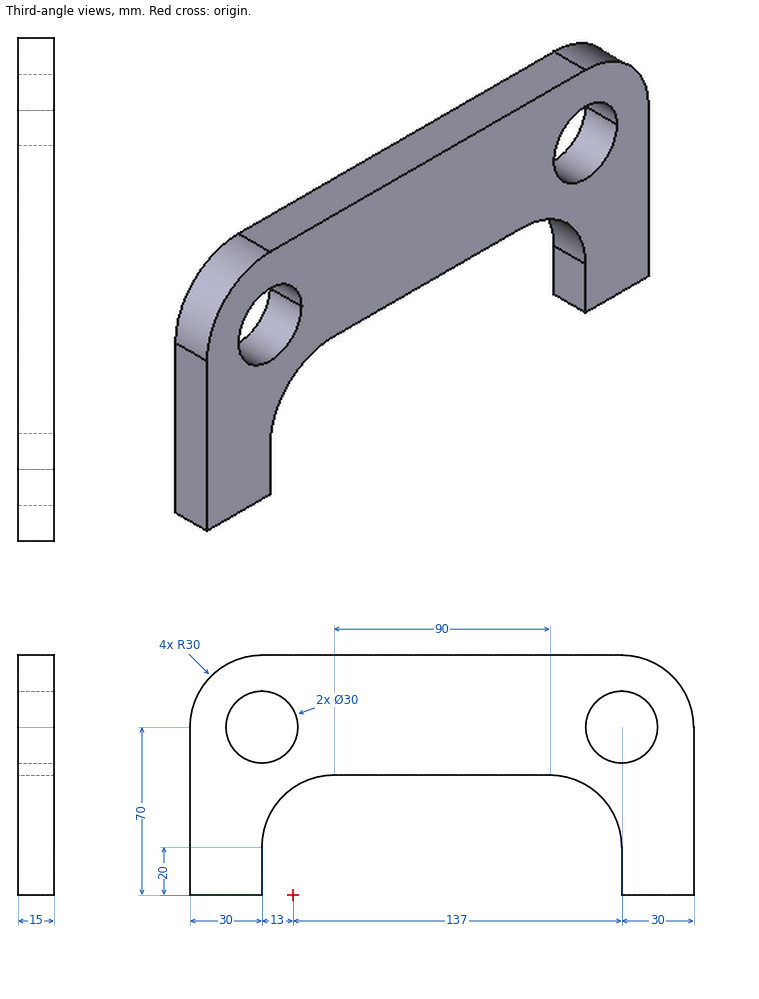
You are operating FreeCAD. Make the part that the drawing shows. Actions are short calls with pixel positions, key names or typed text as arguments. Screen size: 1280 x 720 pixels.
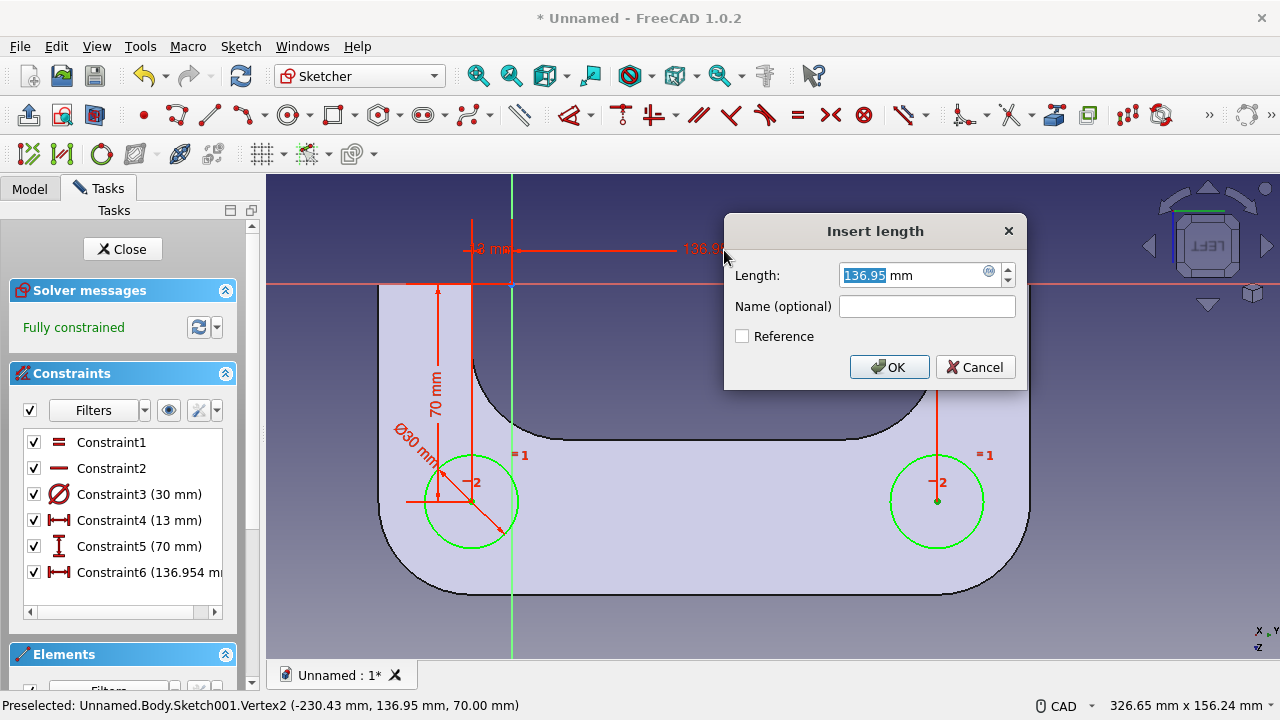
text(137)
key(Return)
key(Escape)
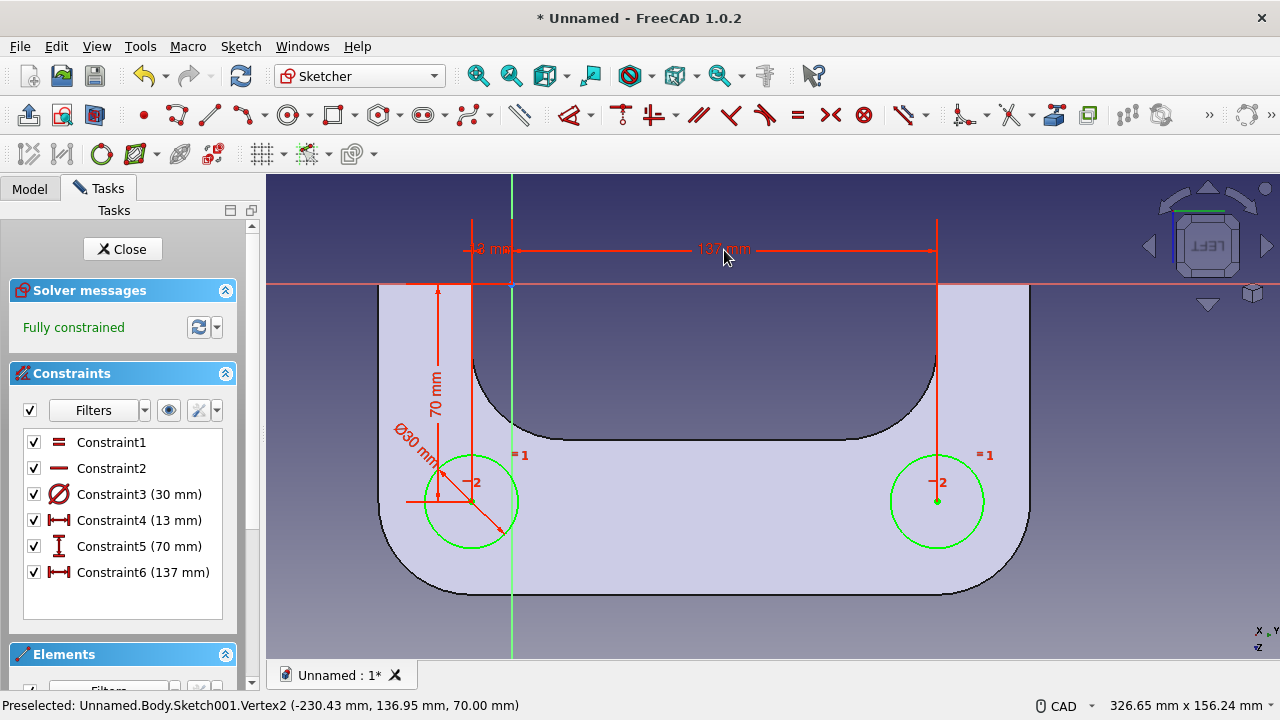
click(123, 249)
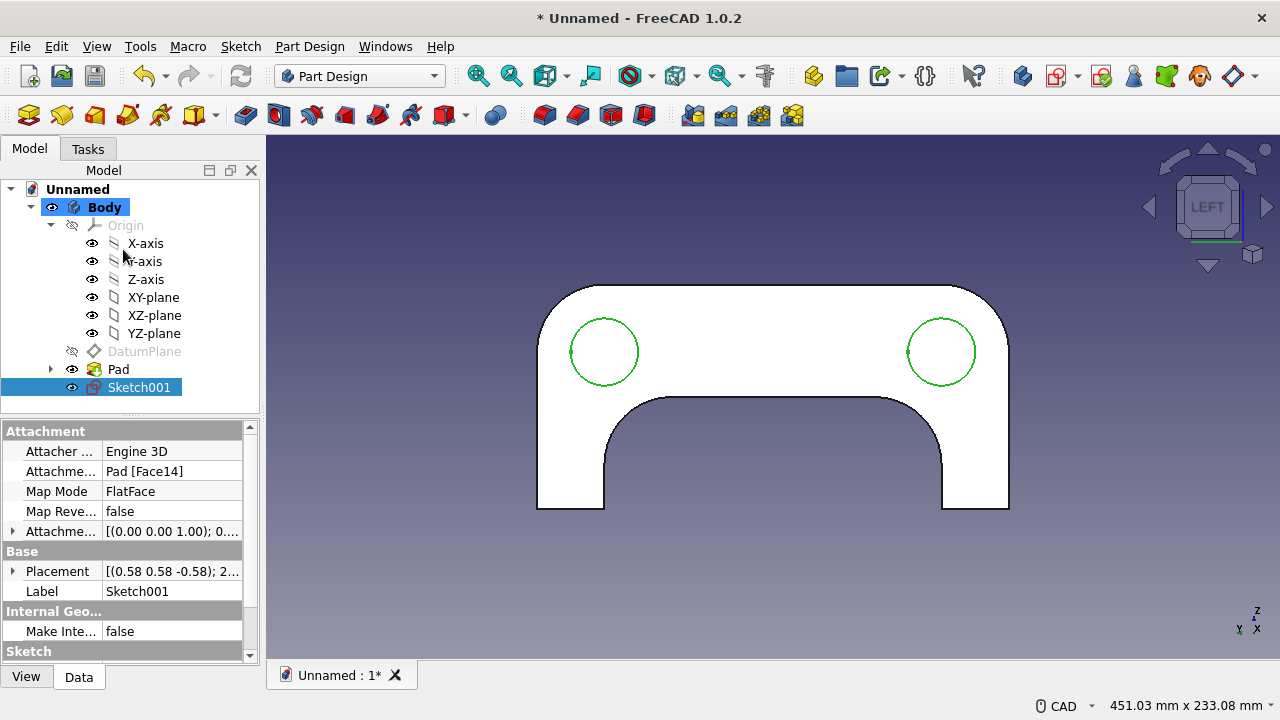
click(246, 116)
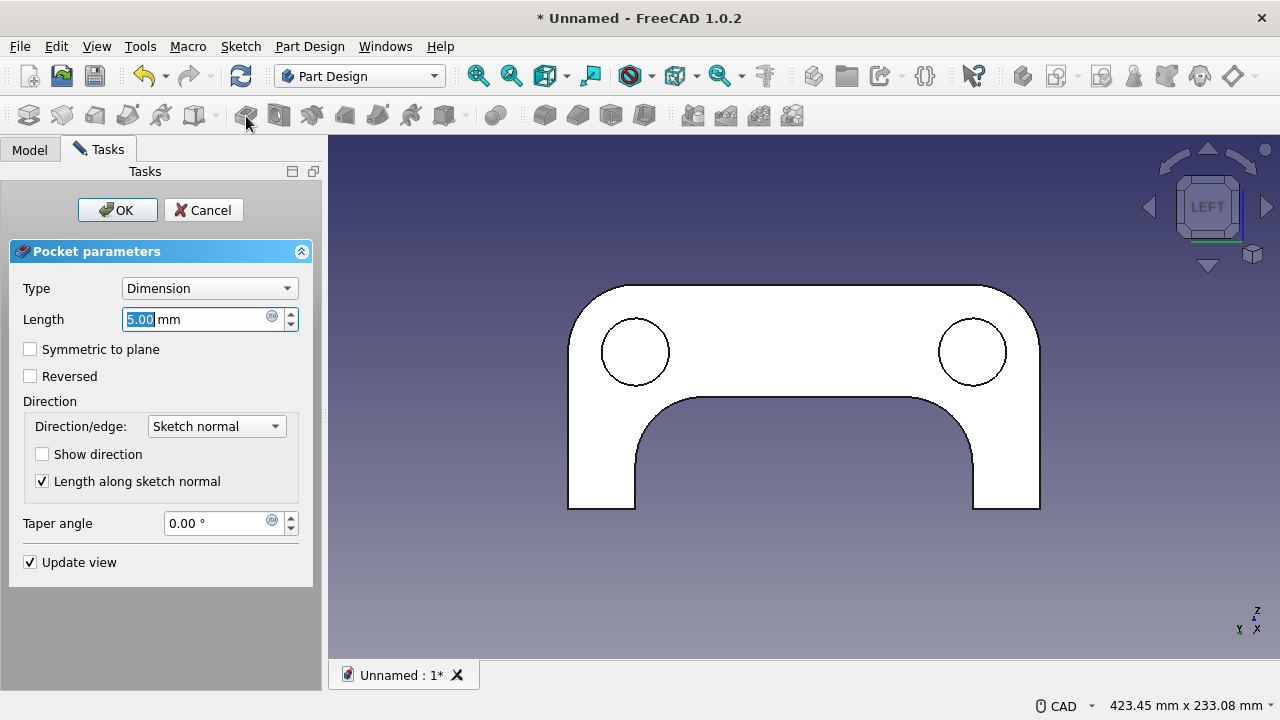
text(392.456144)
key(Tab)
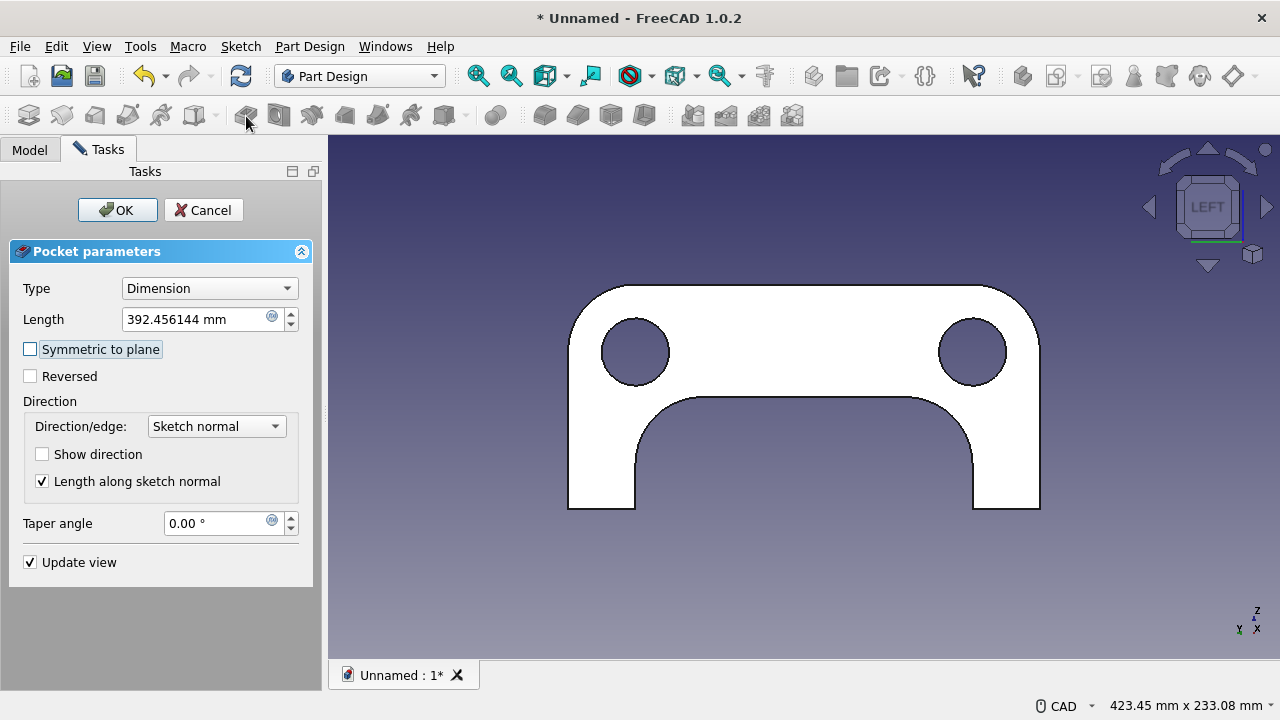
click(31, 349)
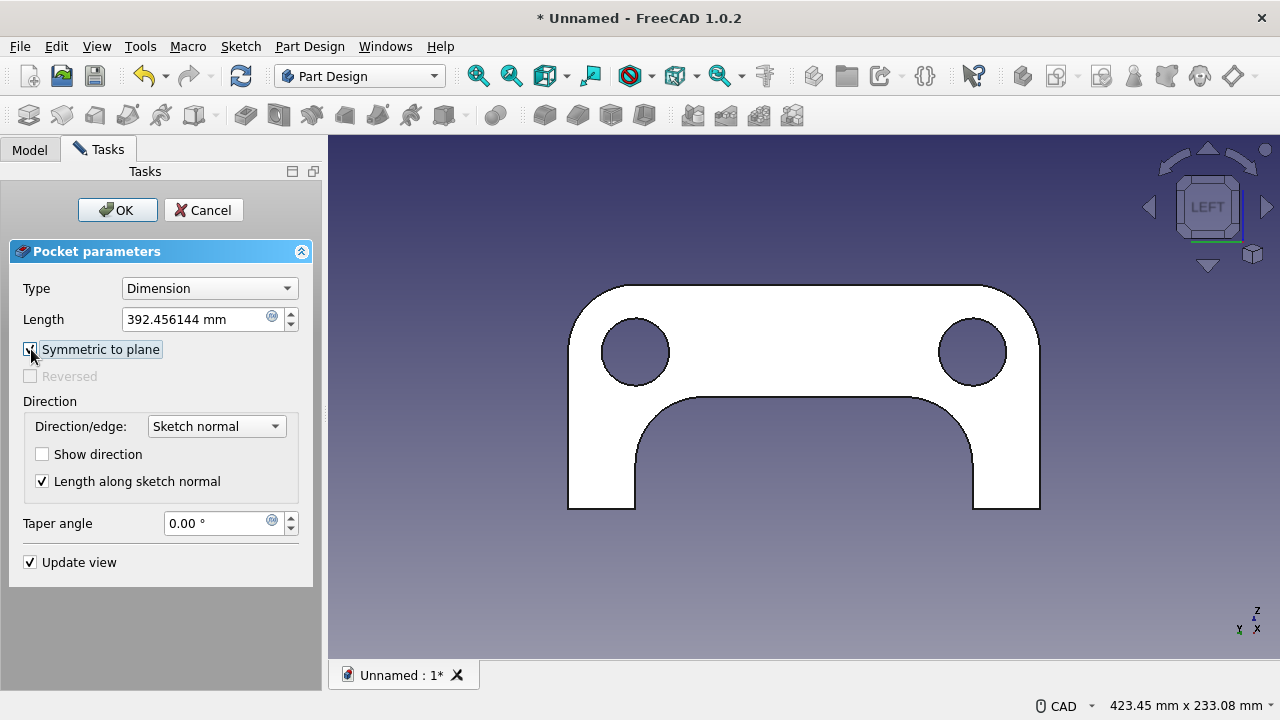
click(118, 210)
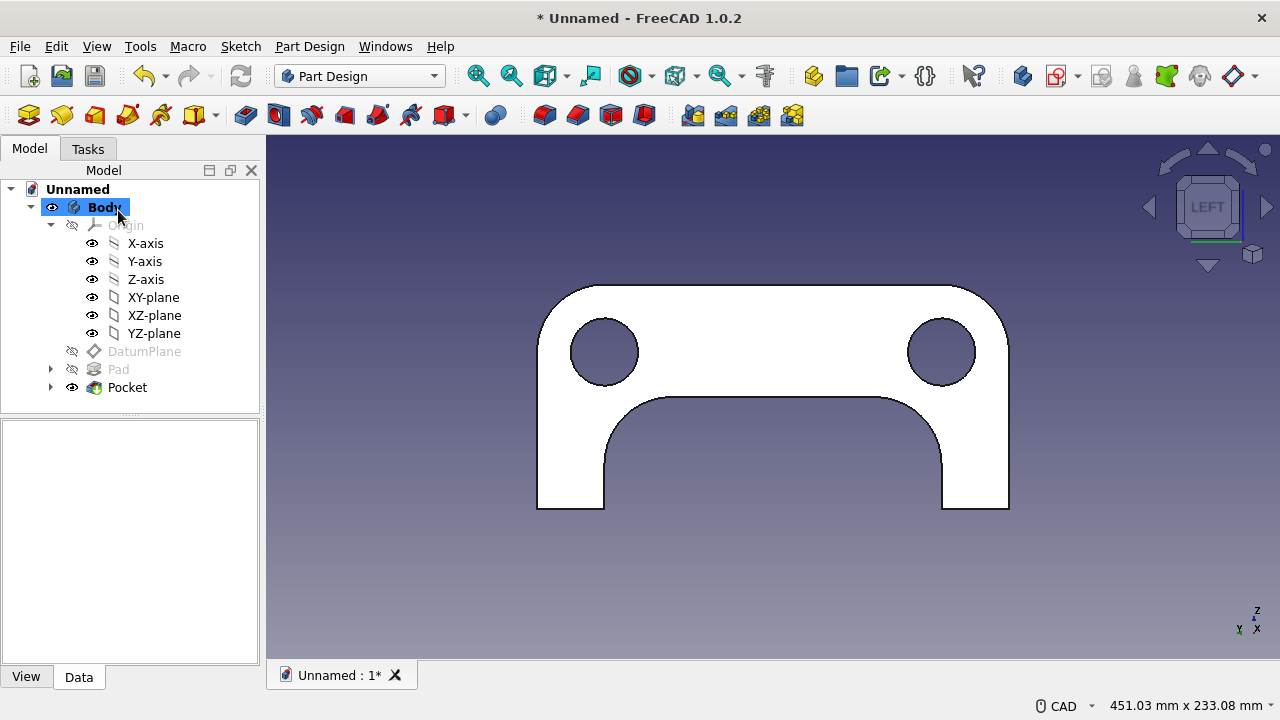
key(0)